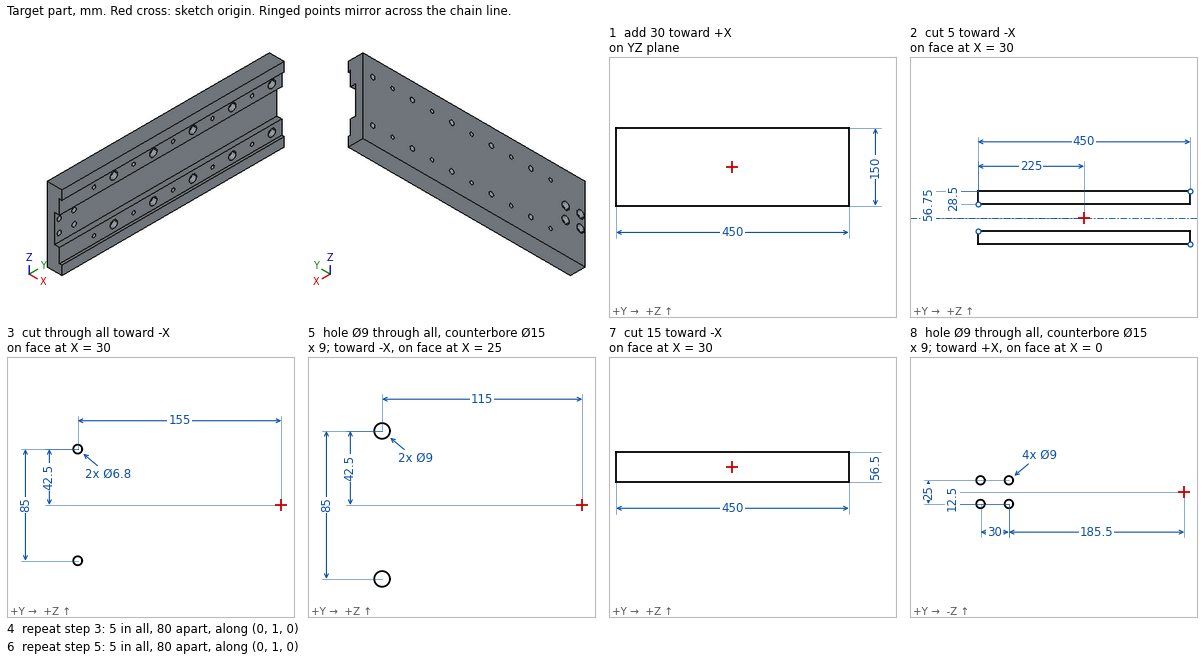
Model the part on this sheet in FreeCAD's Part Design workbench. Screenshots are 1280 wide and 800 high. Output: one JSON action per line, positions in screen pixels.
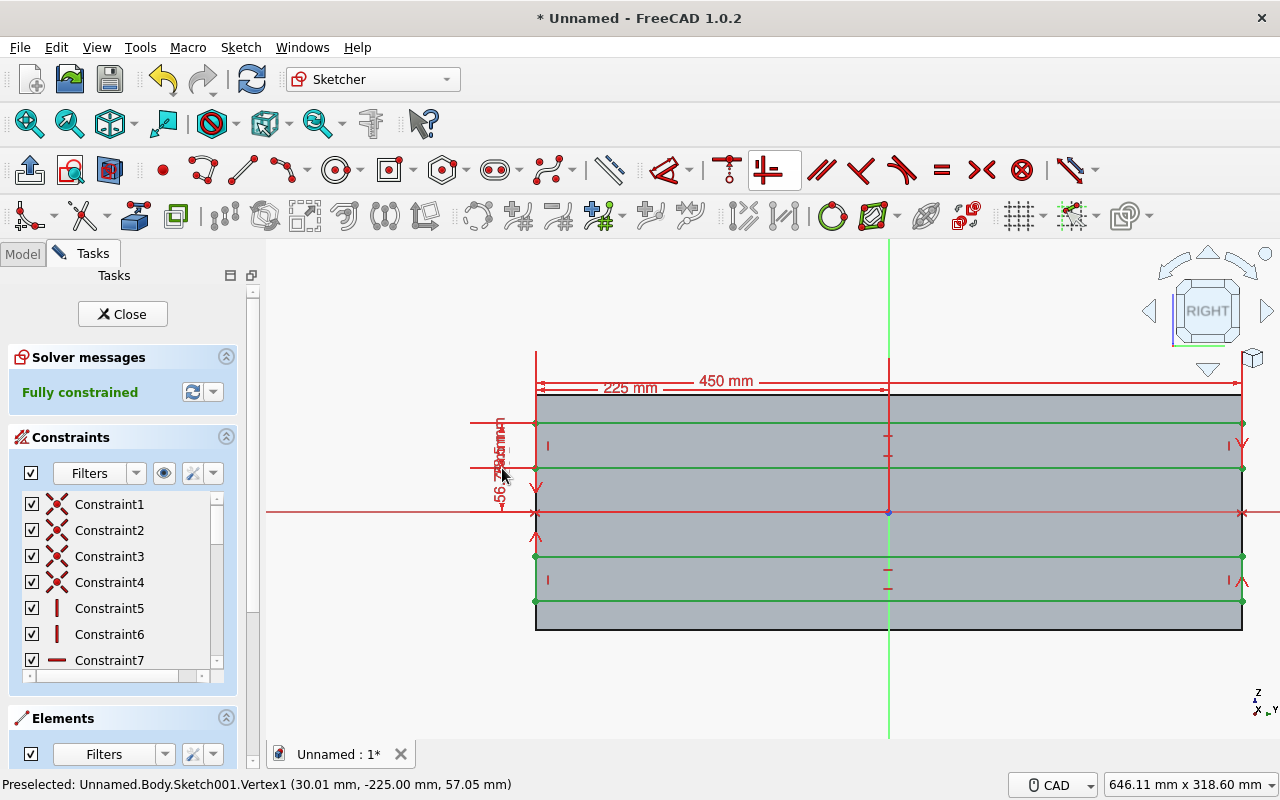
{"action": "left_click", "coordinate": [123, 314]}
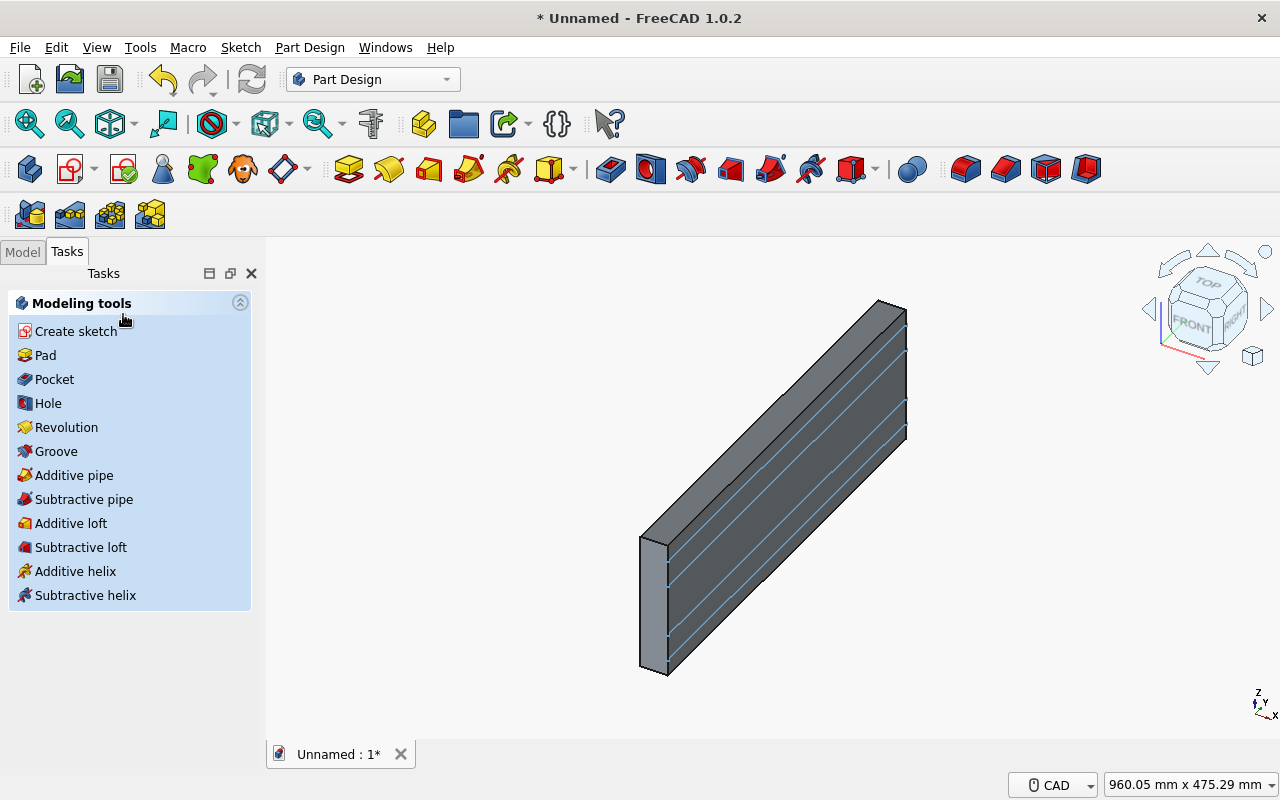
{"action": "left_click", "coordinate": [612, 170]}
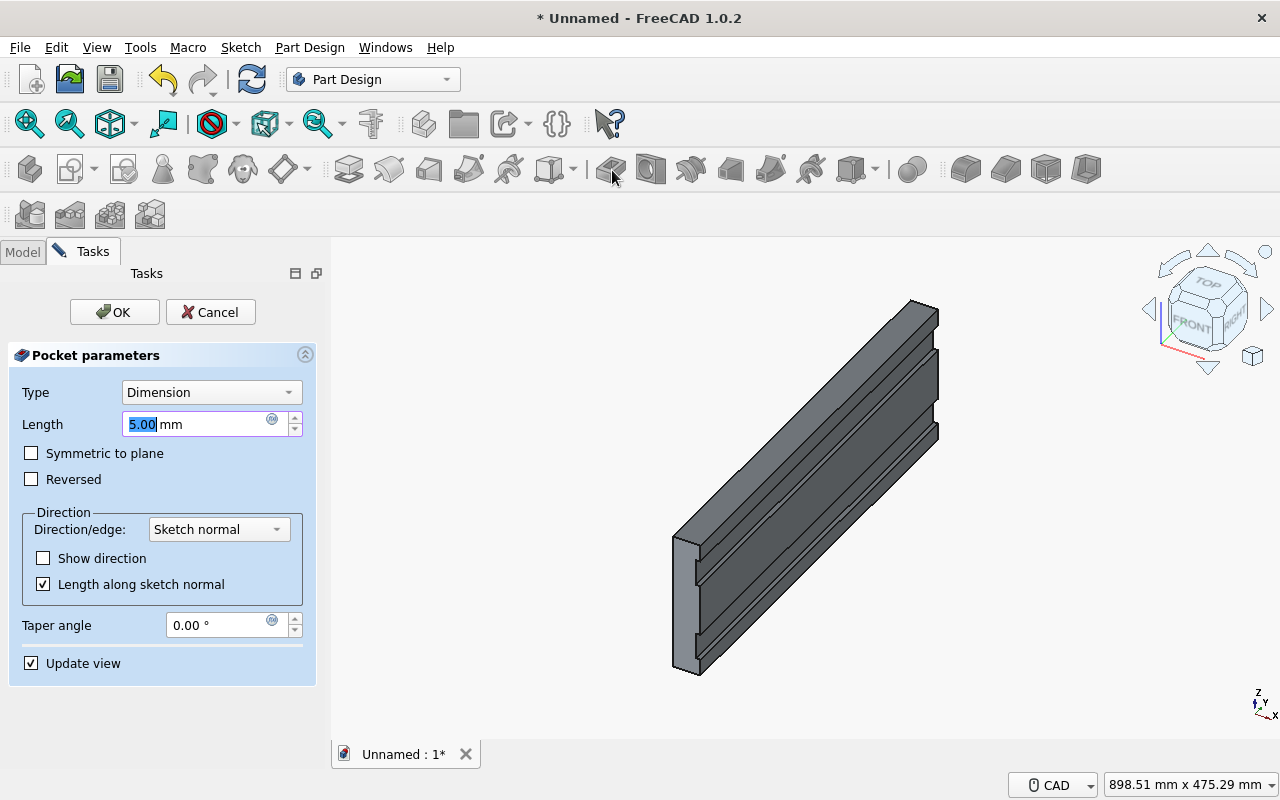
{"action": "type", "text": "5"}
{"action": "key", "text": "Tab"}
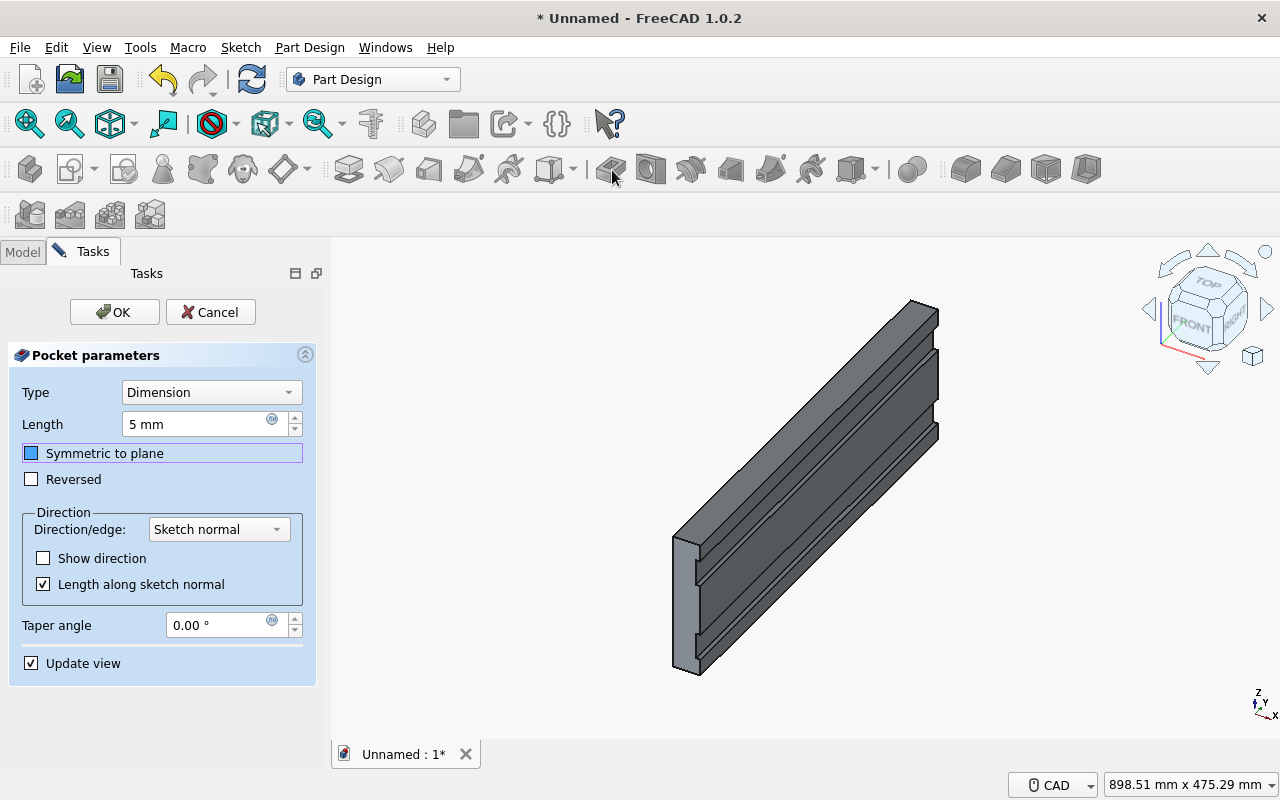
{"action": "left_click", "coordinate": [115, 312]}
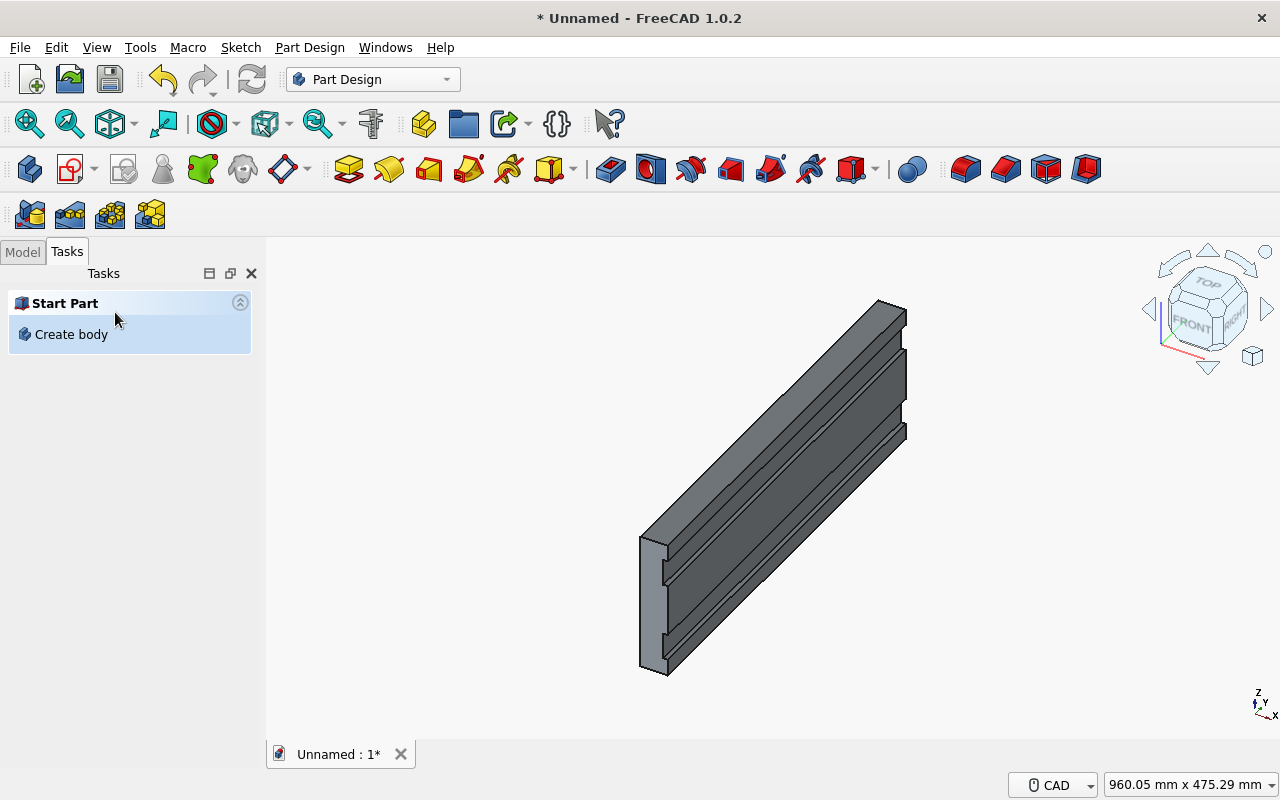
{"action": "left_click", "coordinate": [787, 492]}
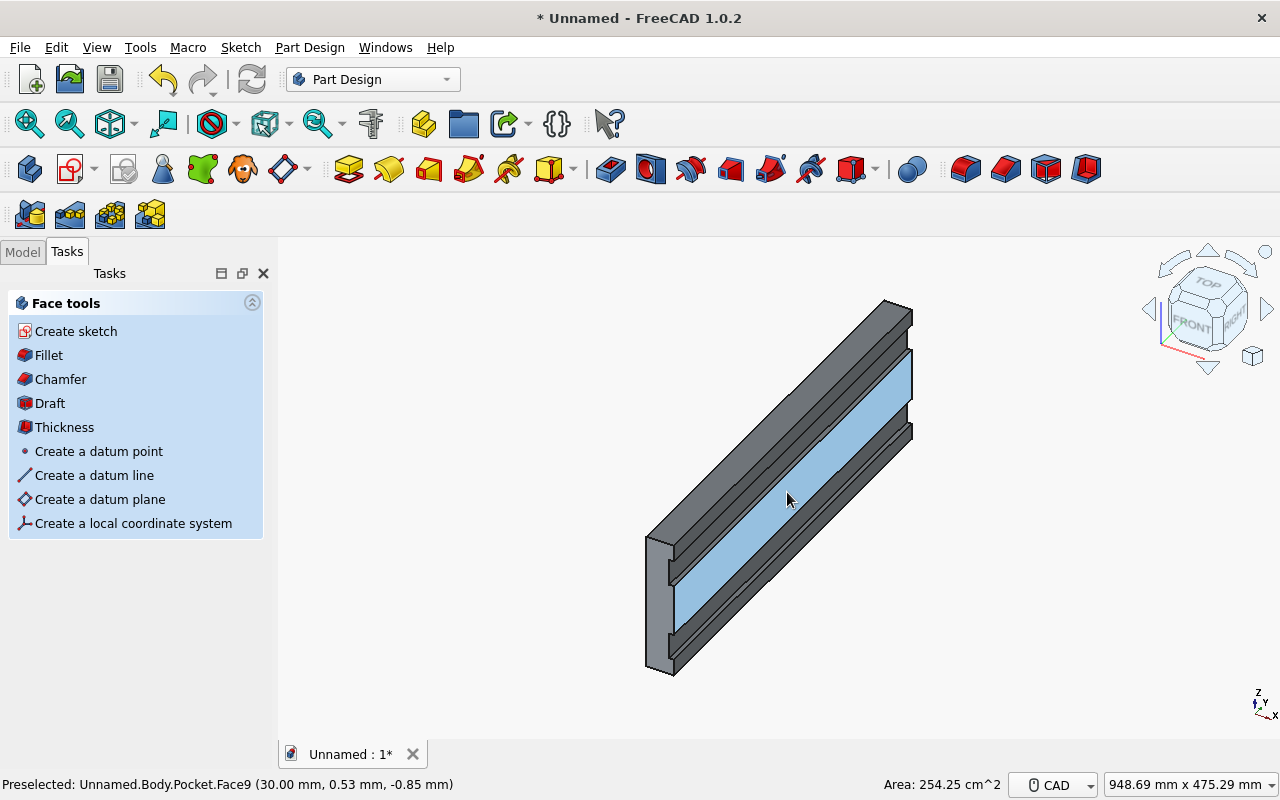
{"action": "left_click", "coordinate": [70, 170]}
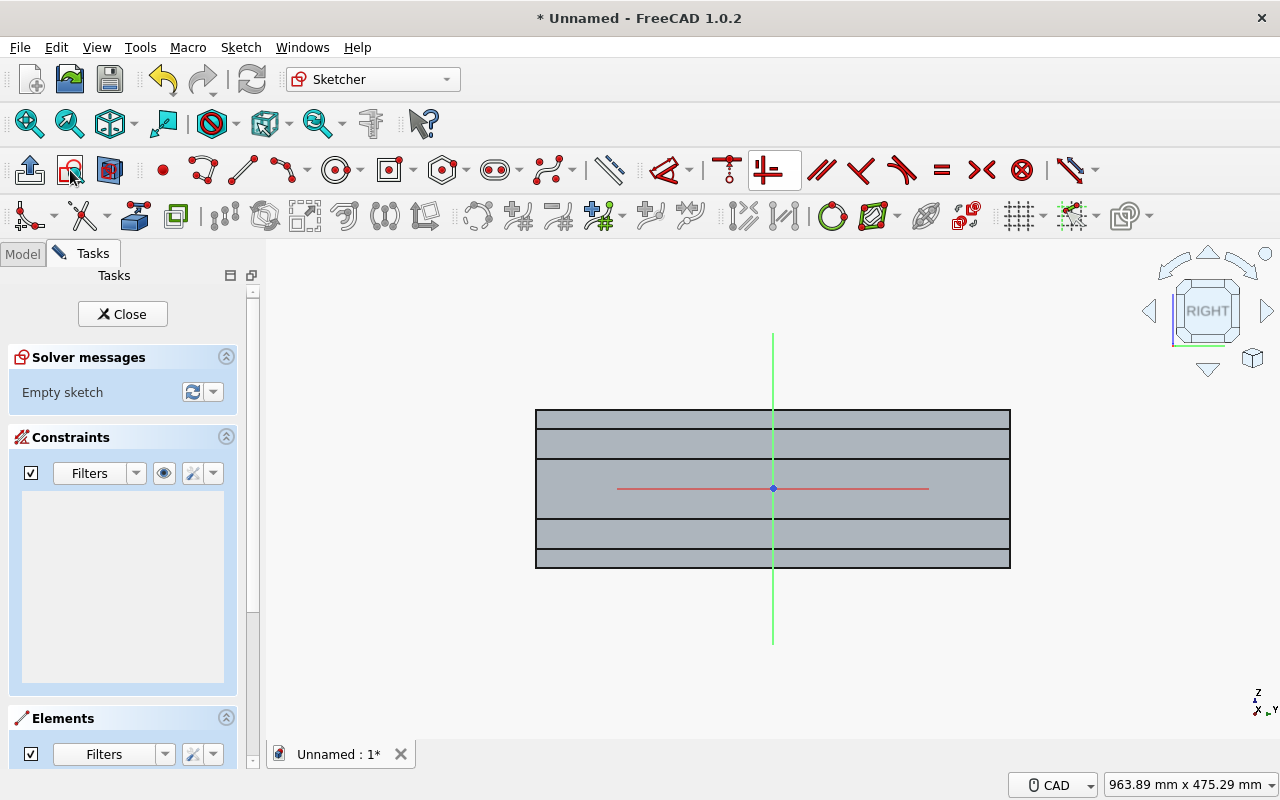
{"action": "scroll", "coordinate": [683, 489], "scroll_direction": "up", "scroll_amount": 6}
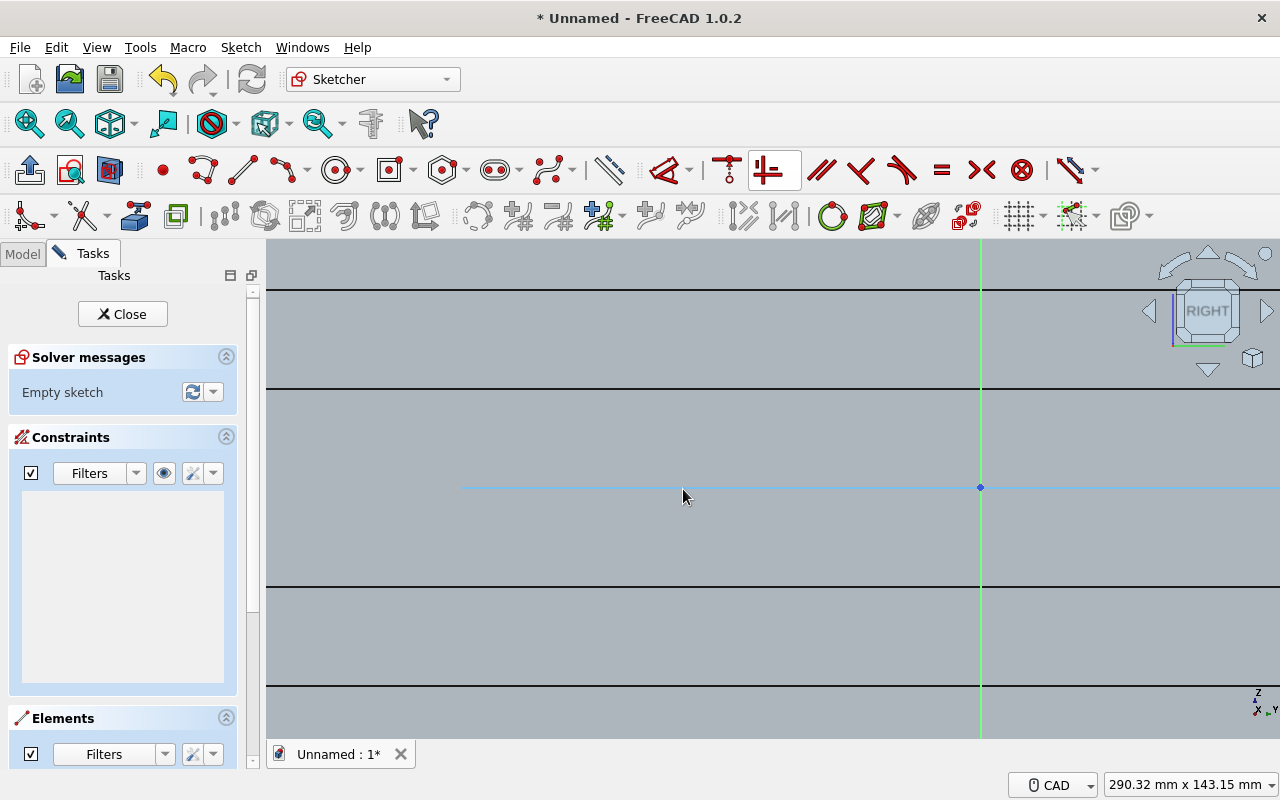
{"action": "left_click", "coordinate": [336, 170]}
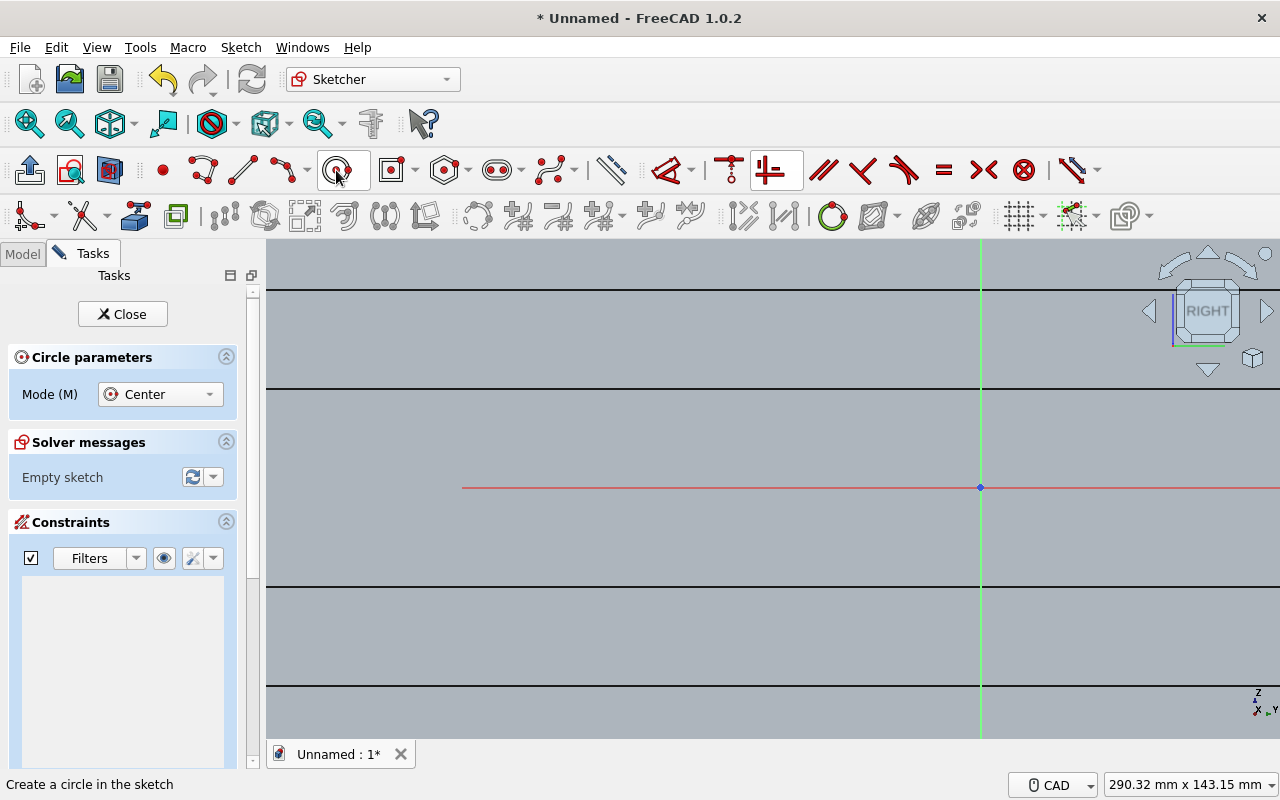
{"action": "scroll", "coordinate": [439, 339], "scroll_direction": "up", "scroll_amount": 4}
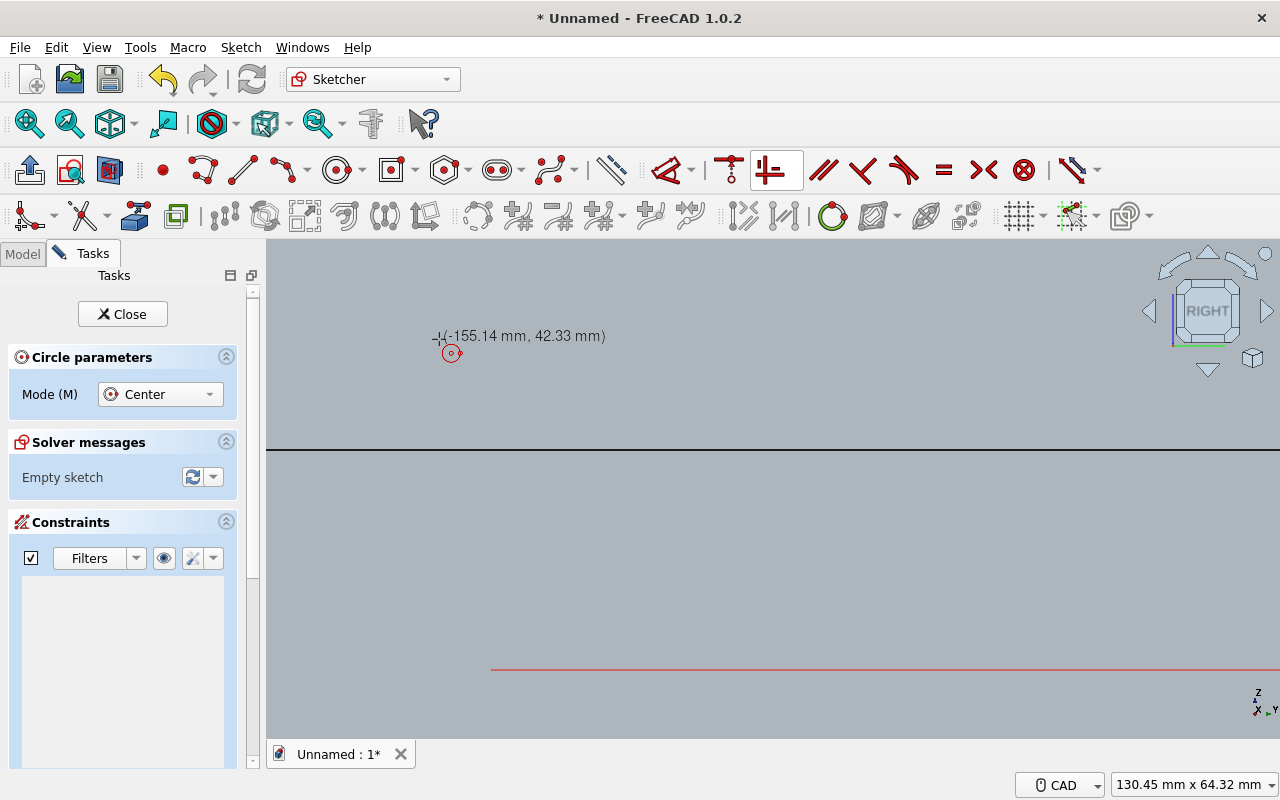
{"action": "left_click", "coordinate": [440, 340]}
{"action": "left_click", "coordinate": [459, 321]}